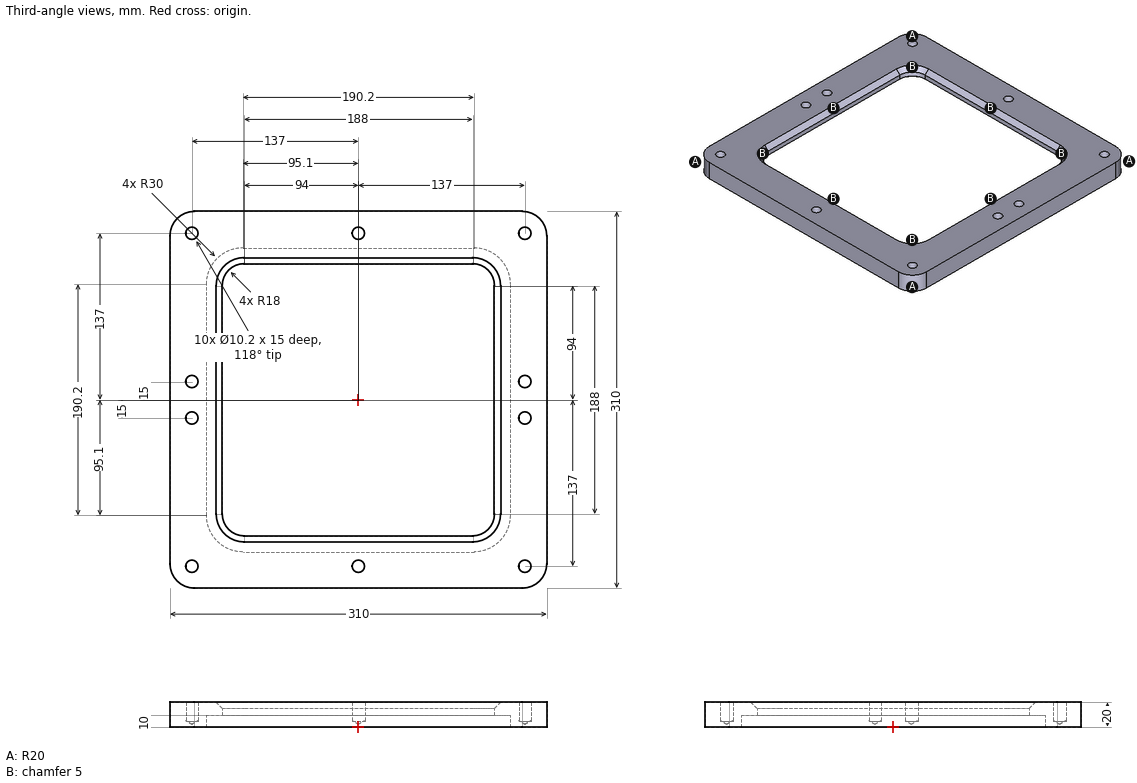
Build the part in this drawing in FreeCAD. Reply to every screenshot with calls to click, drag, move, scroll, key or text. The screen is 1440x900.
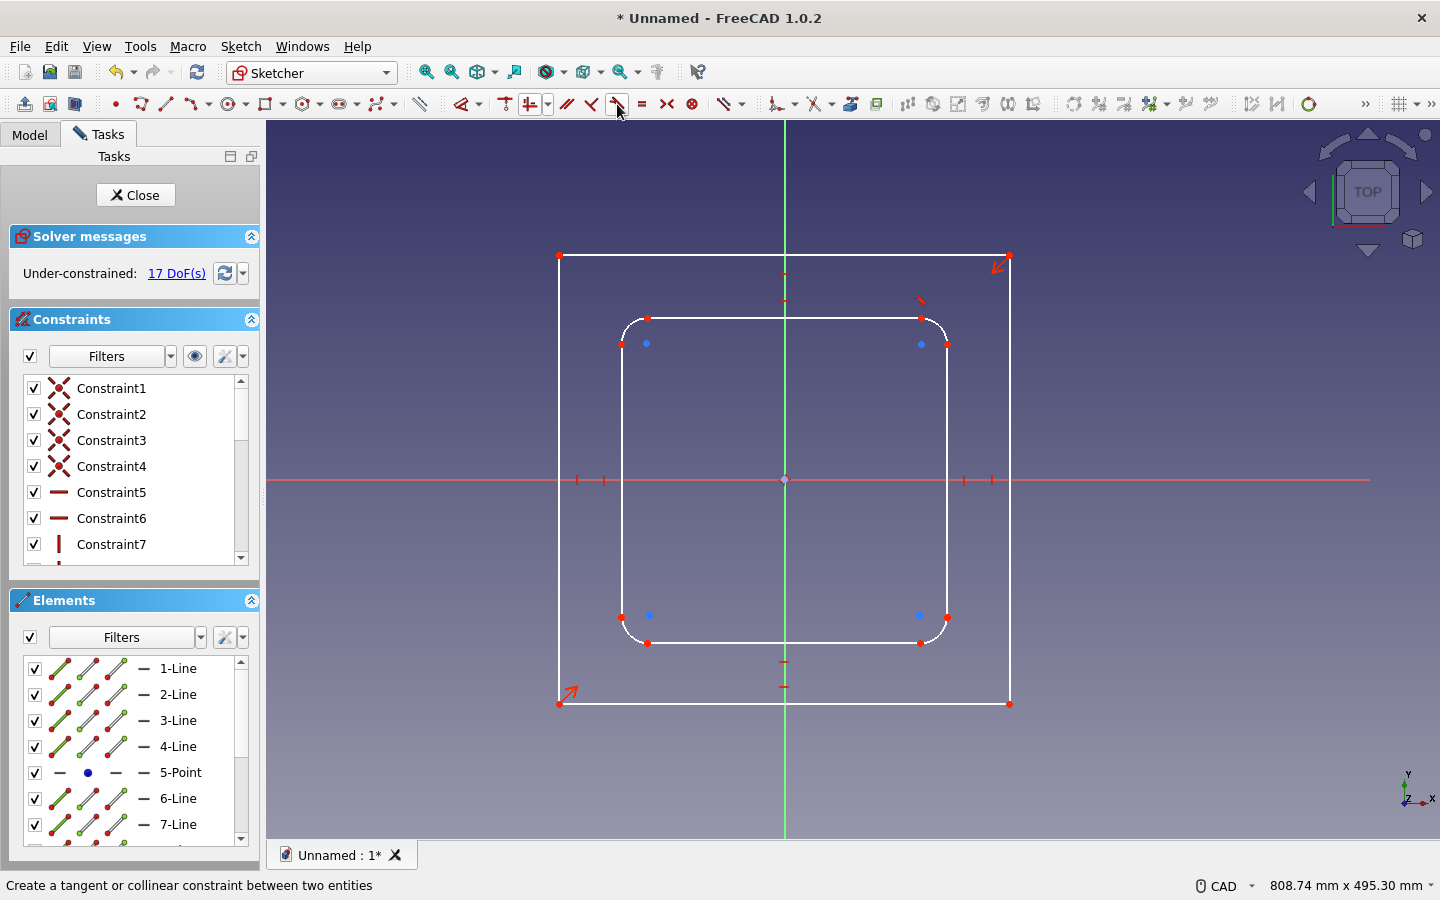
click(730, 318)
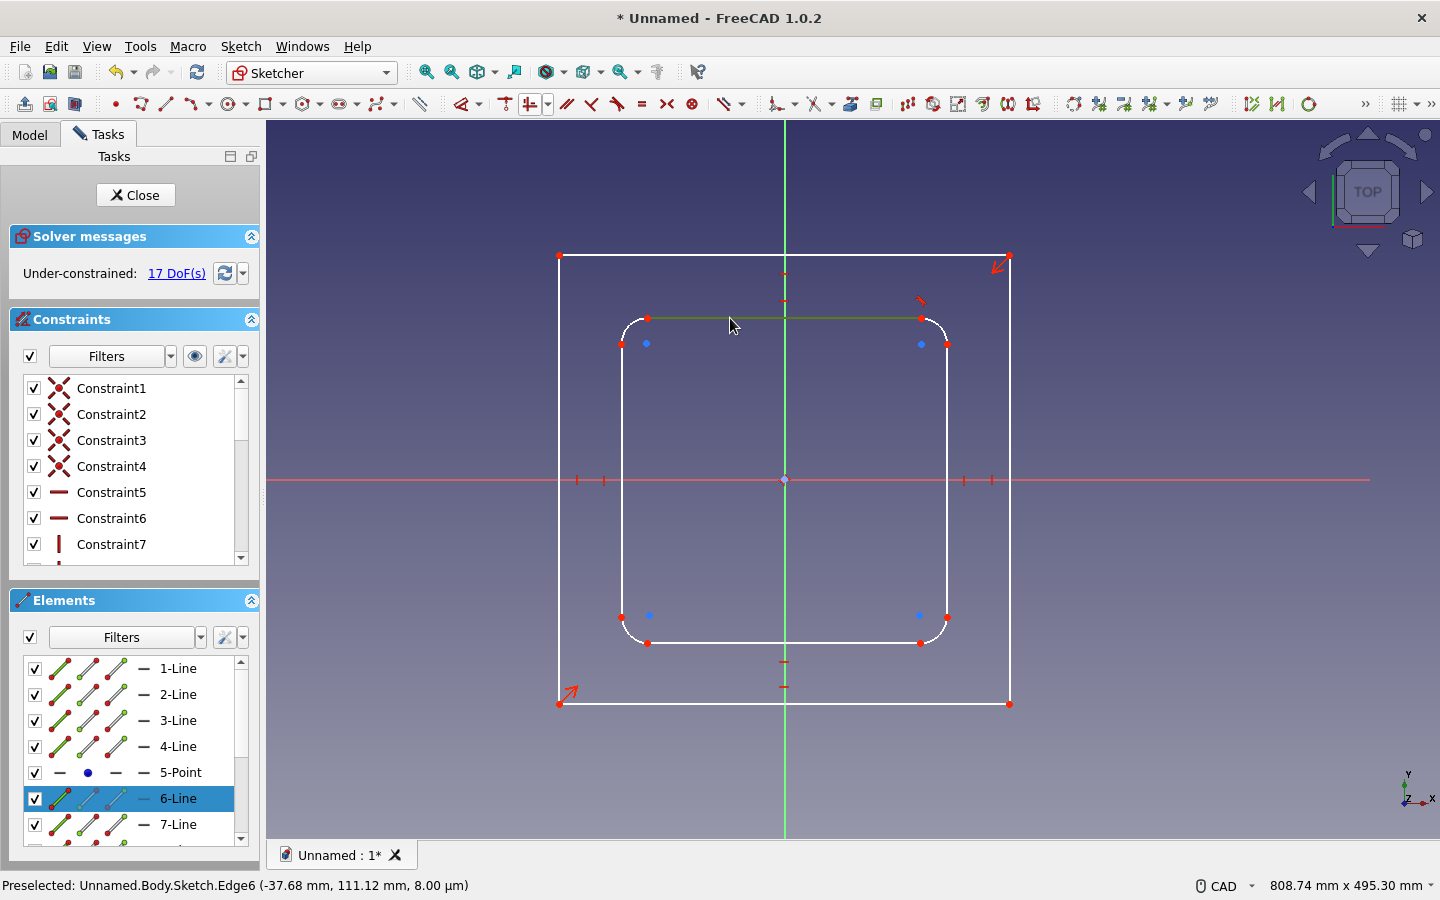
click(636, 321)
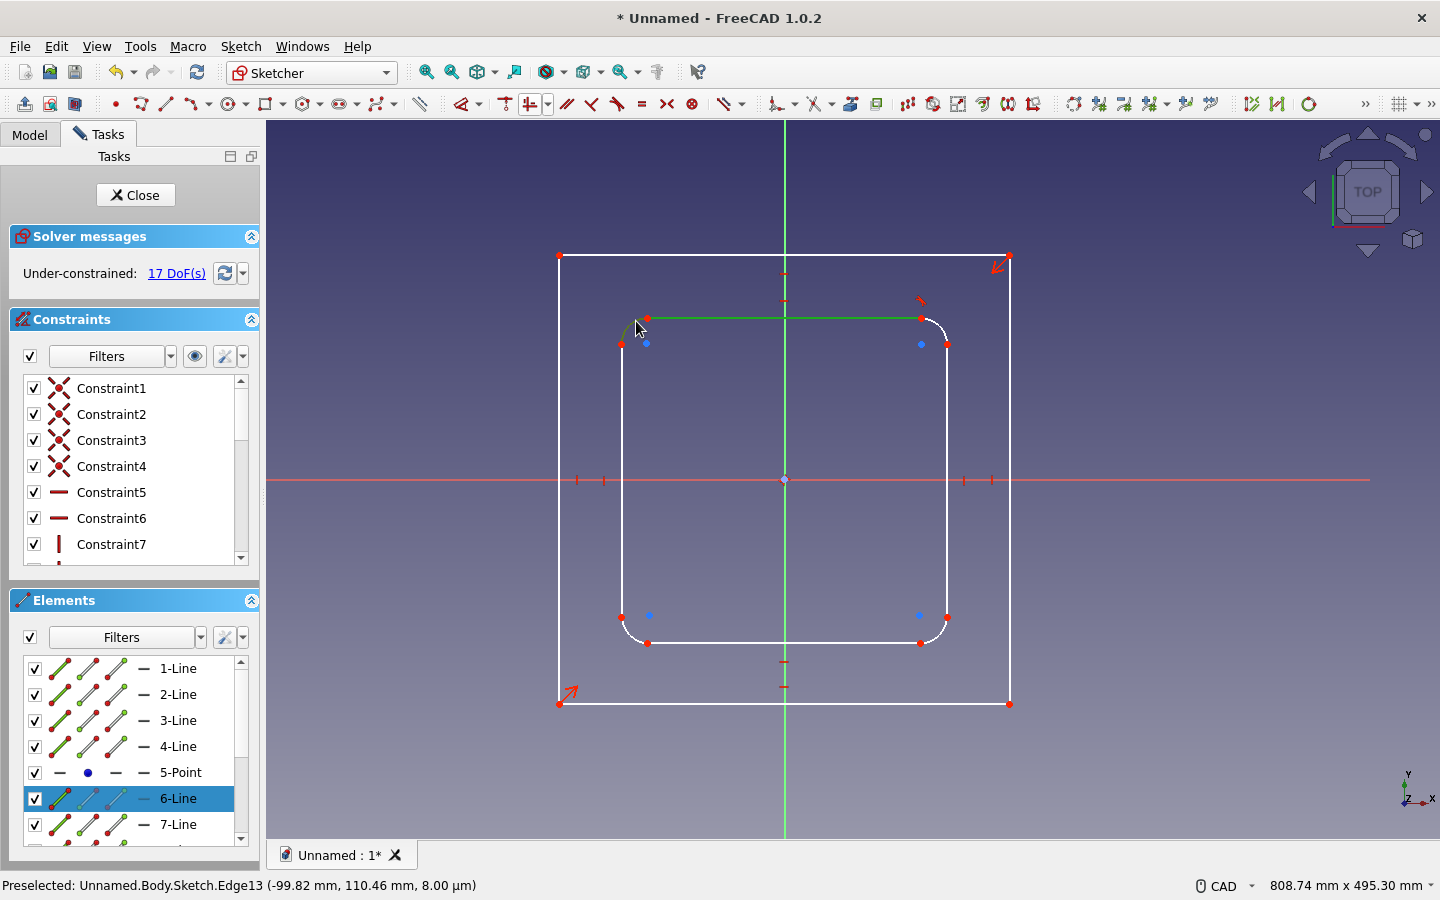
click(617, 104)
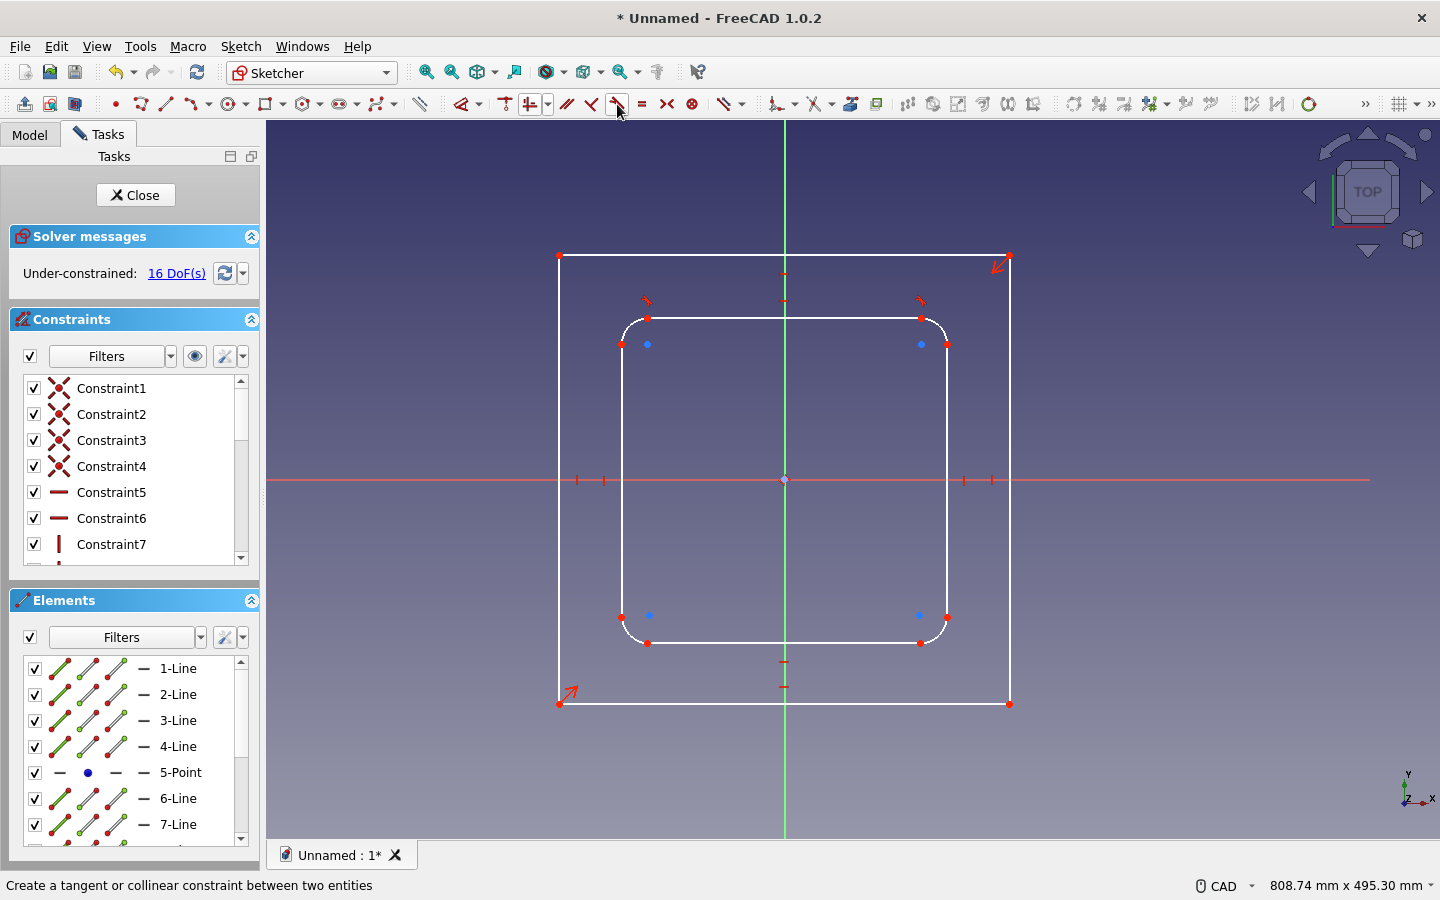
click(947, 426)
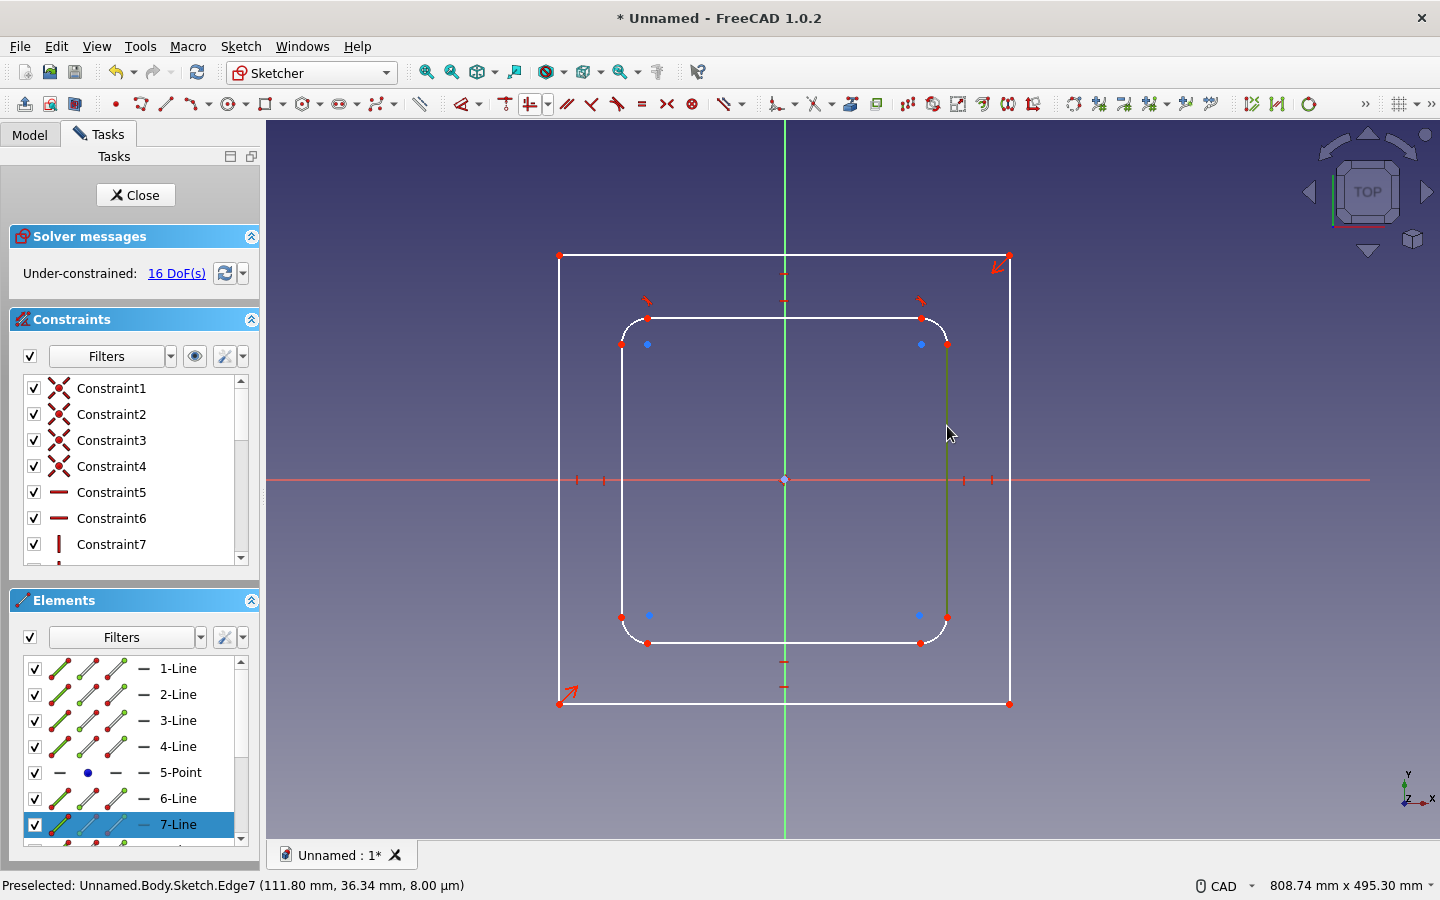
click(944, 333)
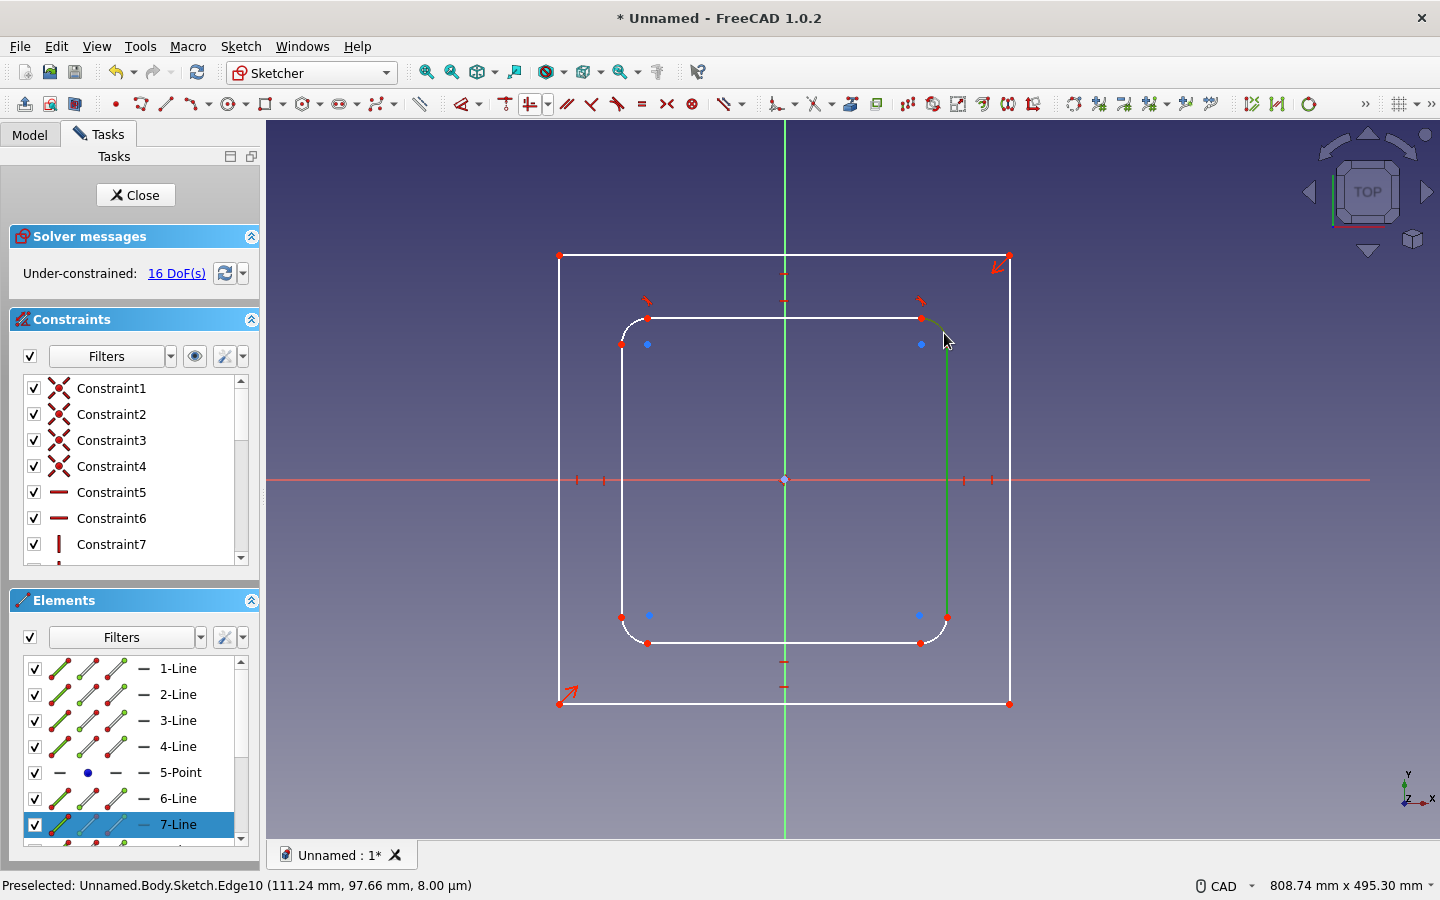
click(617, 104)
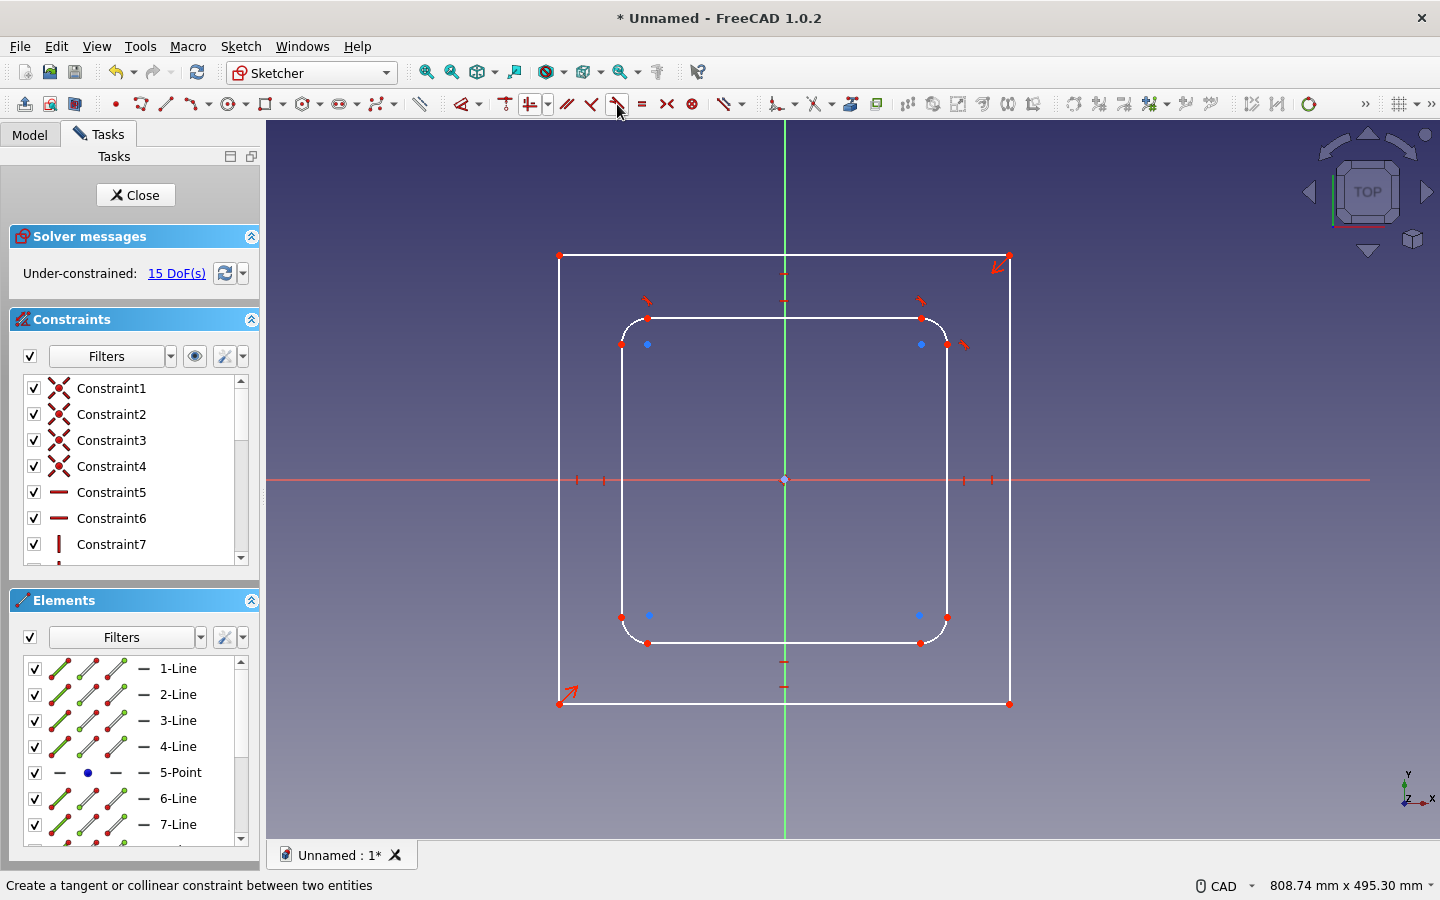
click(947, 426)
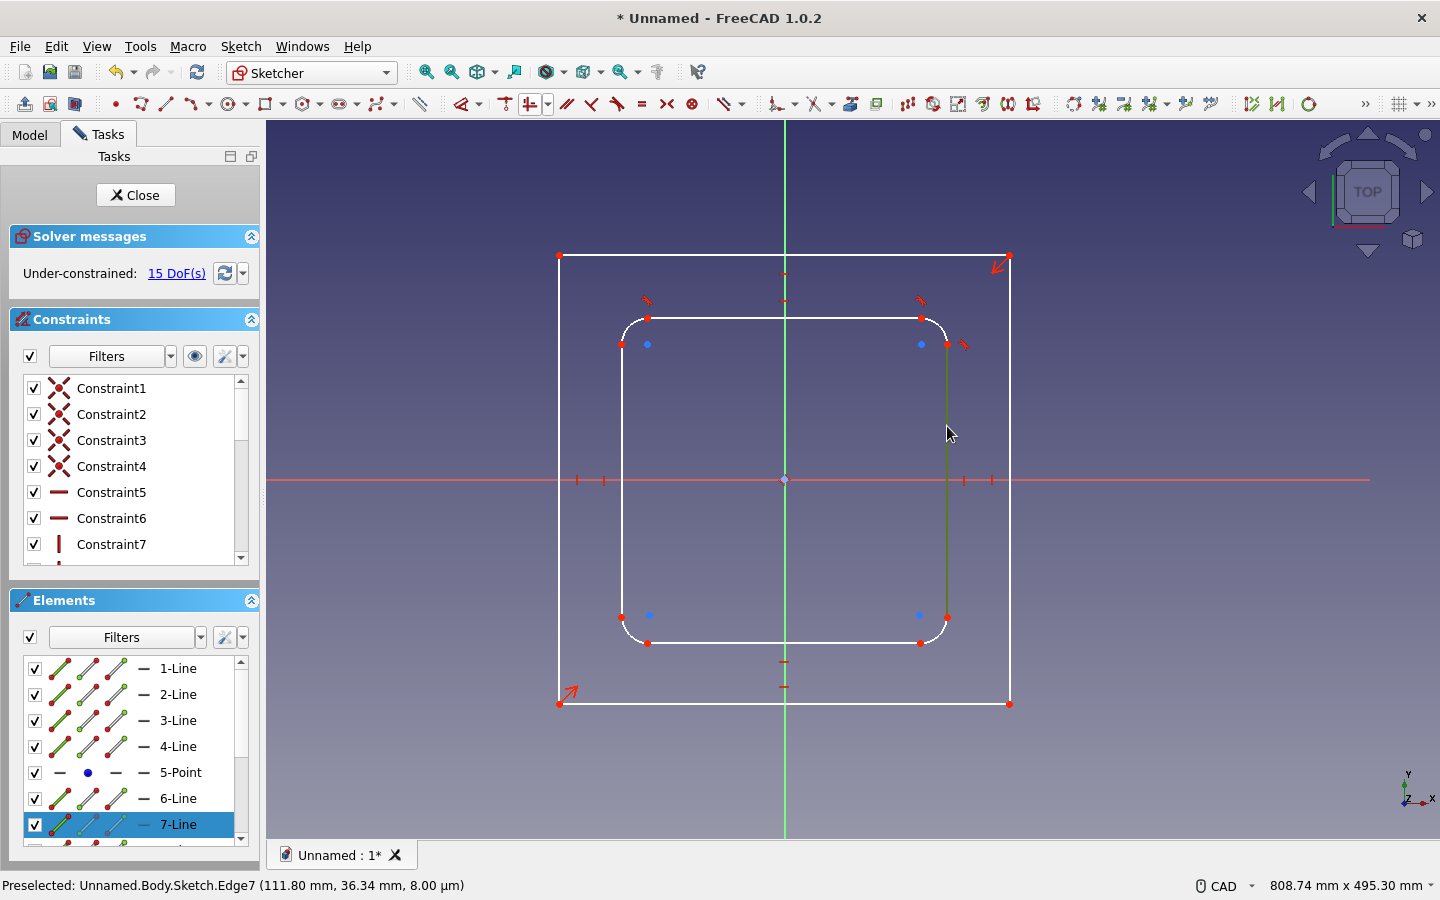
click(933, 640)